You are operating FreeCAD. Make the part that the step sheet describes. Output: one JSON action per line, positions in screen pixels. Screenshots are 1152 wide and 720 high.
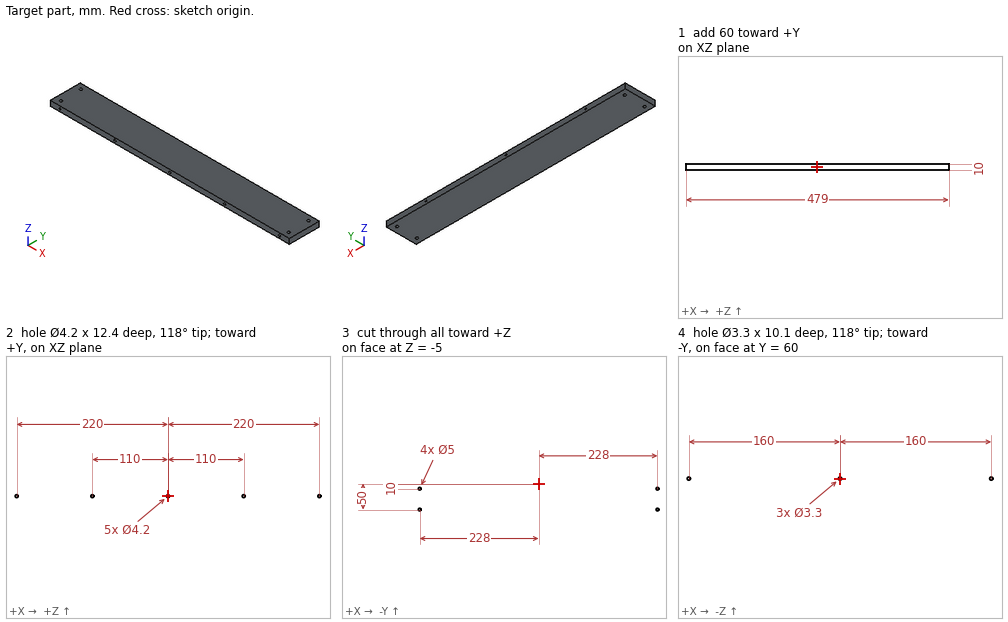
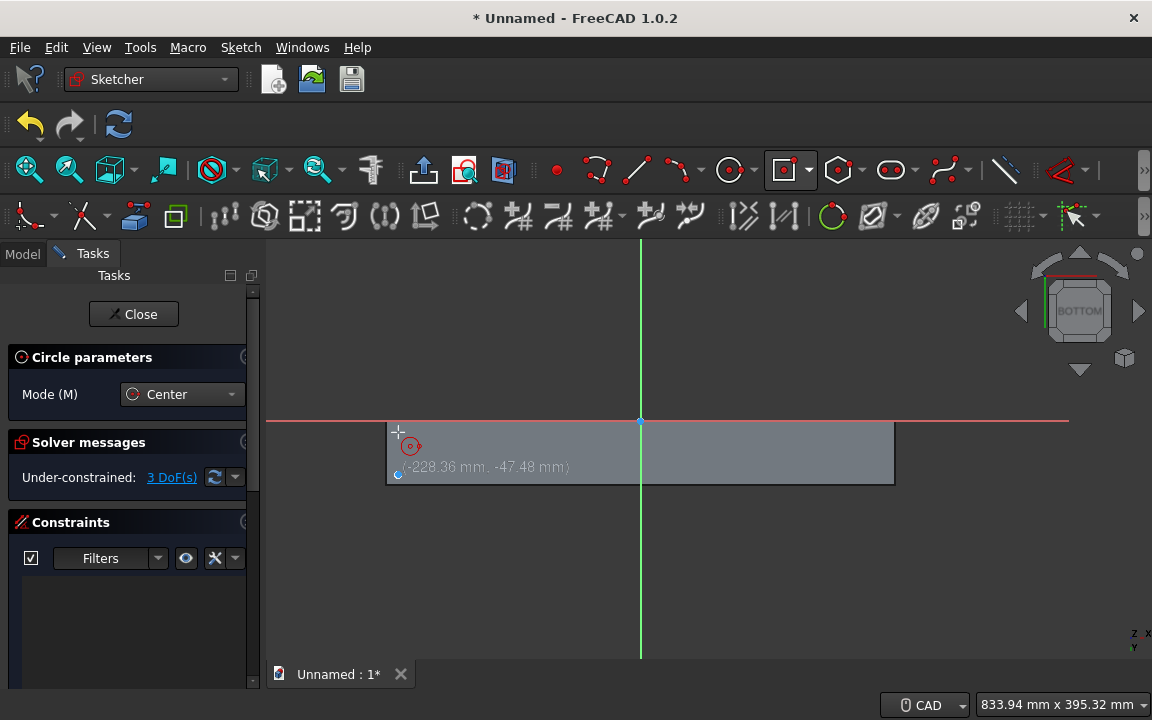
{"action": "scroll", "coordinate": [398, 432], "scroll_direction": "up", "scroll_amount": 3}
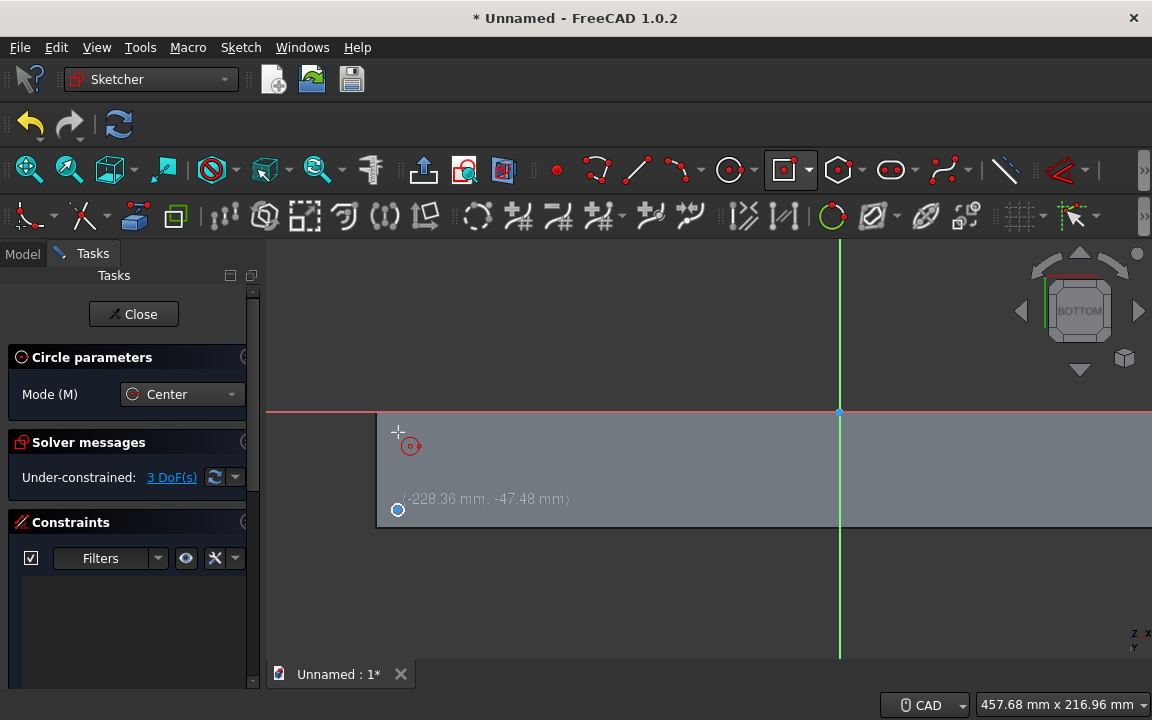
{"action": "left_click", "coordinate": [399, 431]}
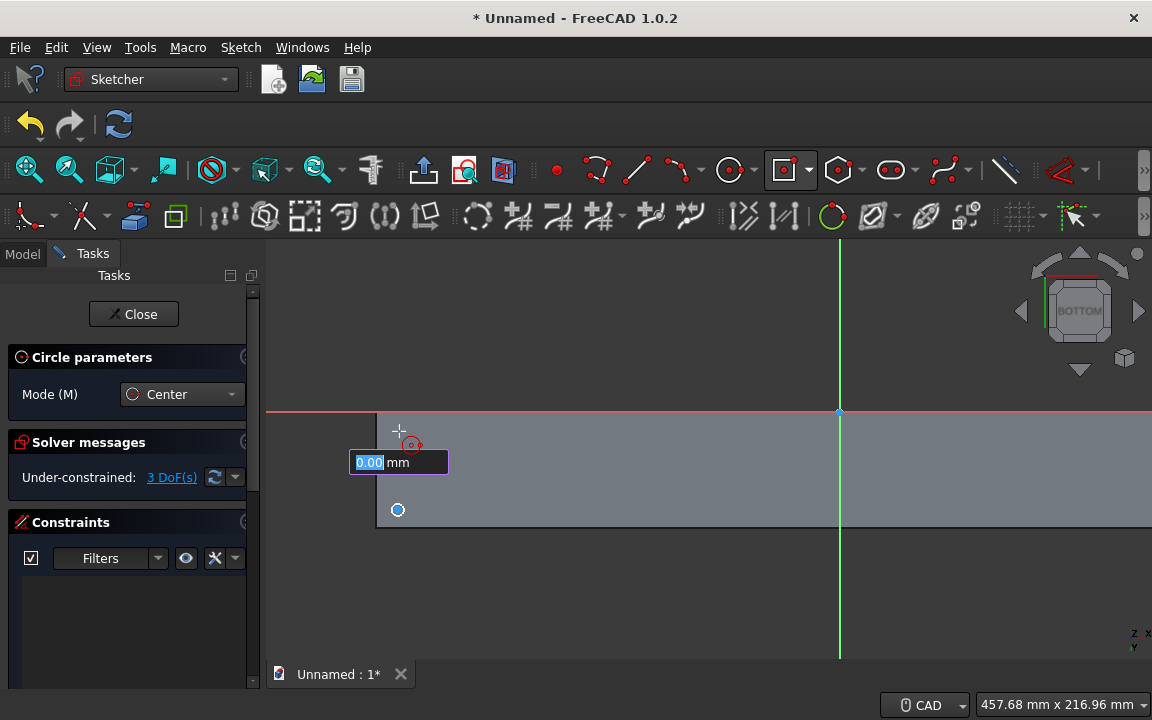
{"action": "scroll", "coordinate": [402, 428], "scroll_direction": "up", "scroll_amount": 6}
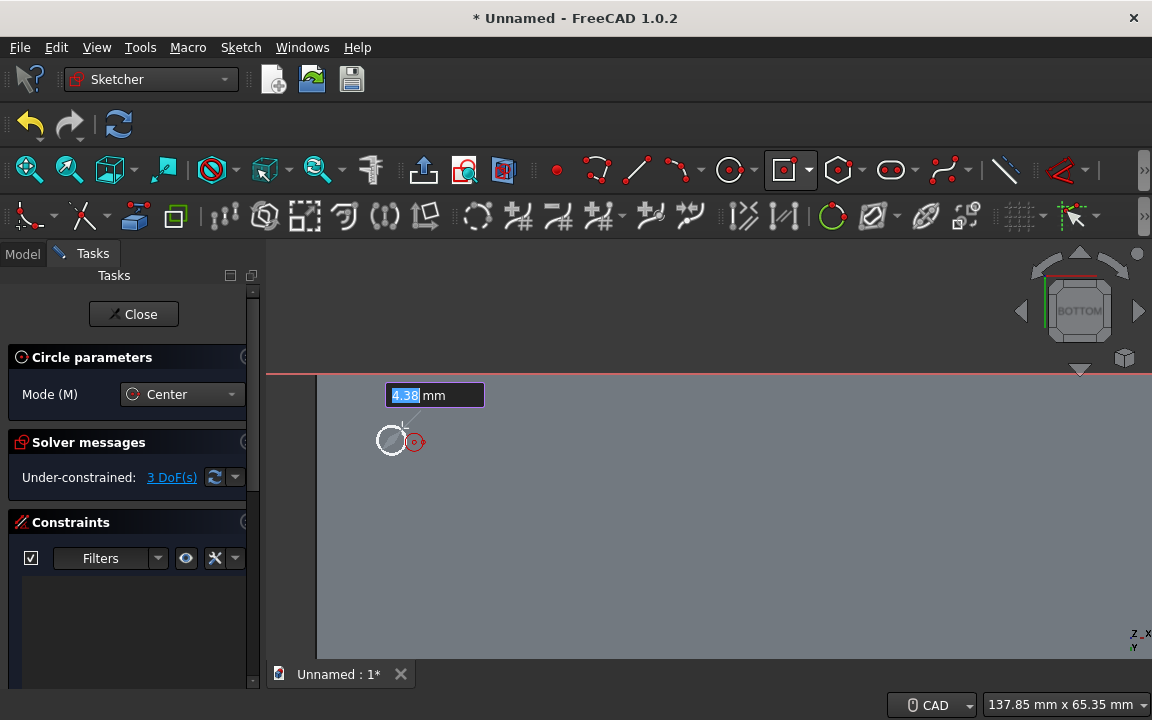
{"action": "left_click", "coordinate": [402, 427]}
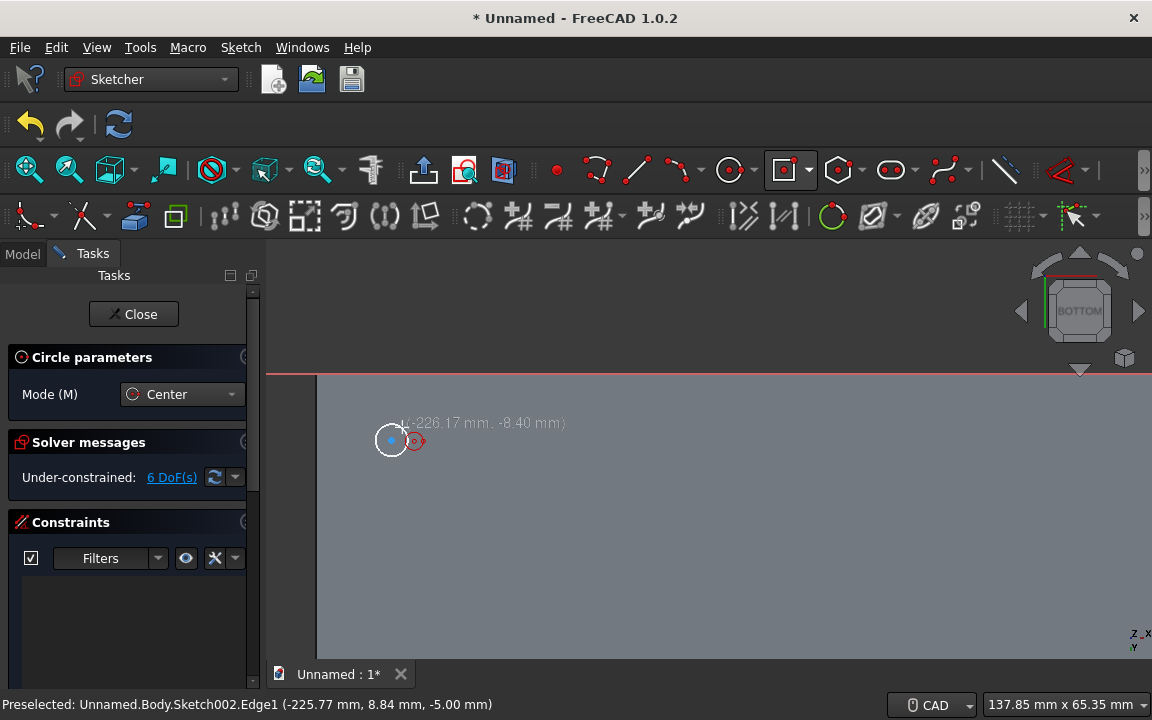
{"action": "scroll", "coordinate": [400, 430], "scroll_direction": "down", "scroll_amount": 9}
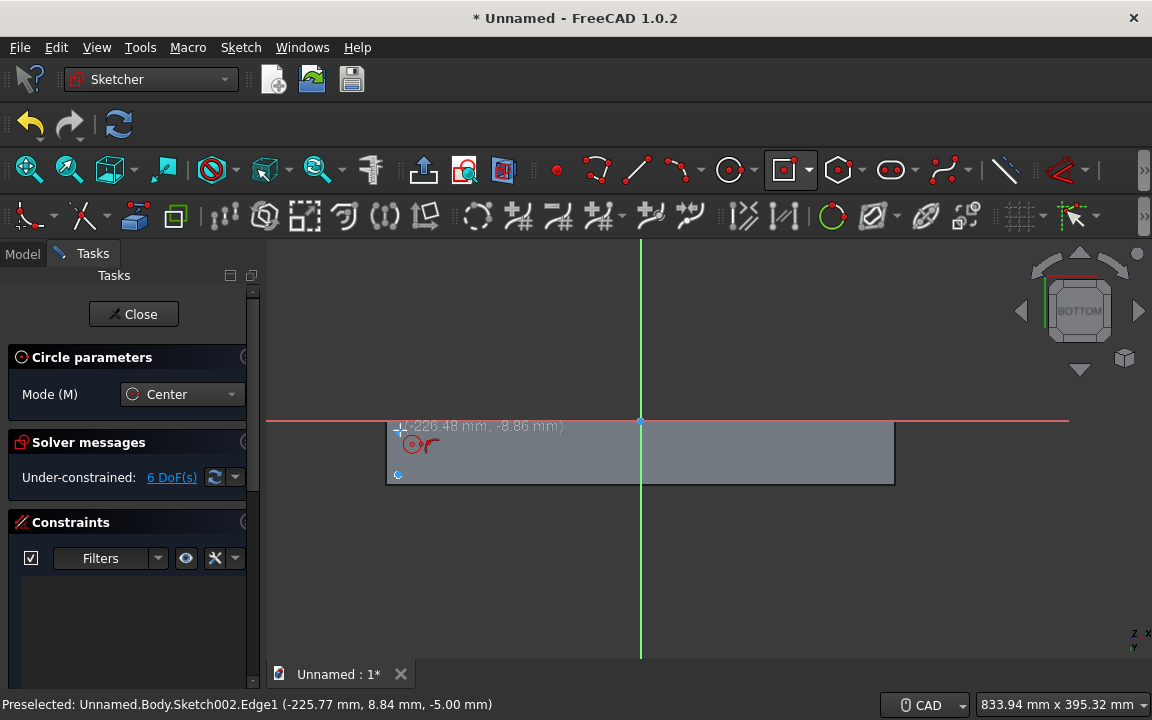
{"action": "scroll", "coordinate": [883, 432], "scroll_direction": "up", "scroll_amount": 11}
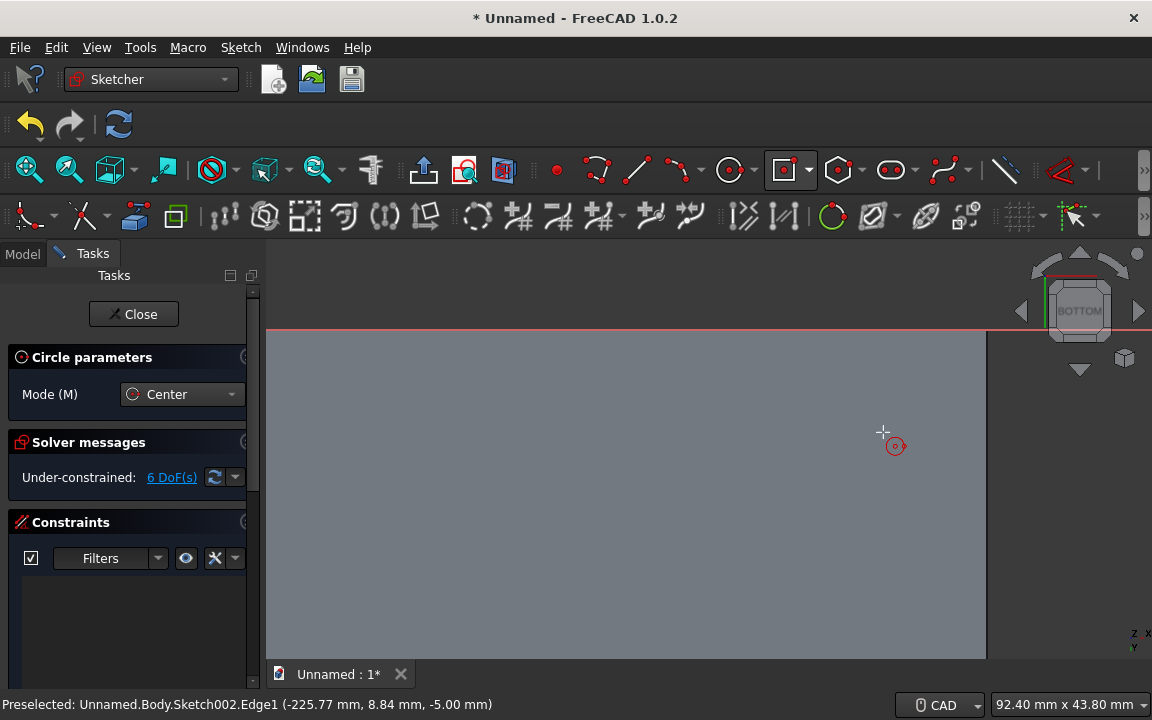
{"action": "scroll", "coordinate": [883, 432], "scroll_direction": "down", "scroll_amount": 11}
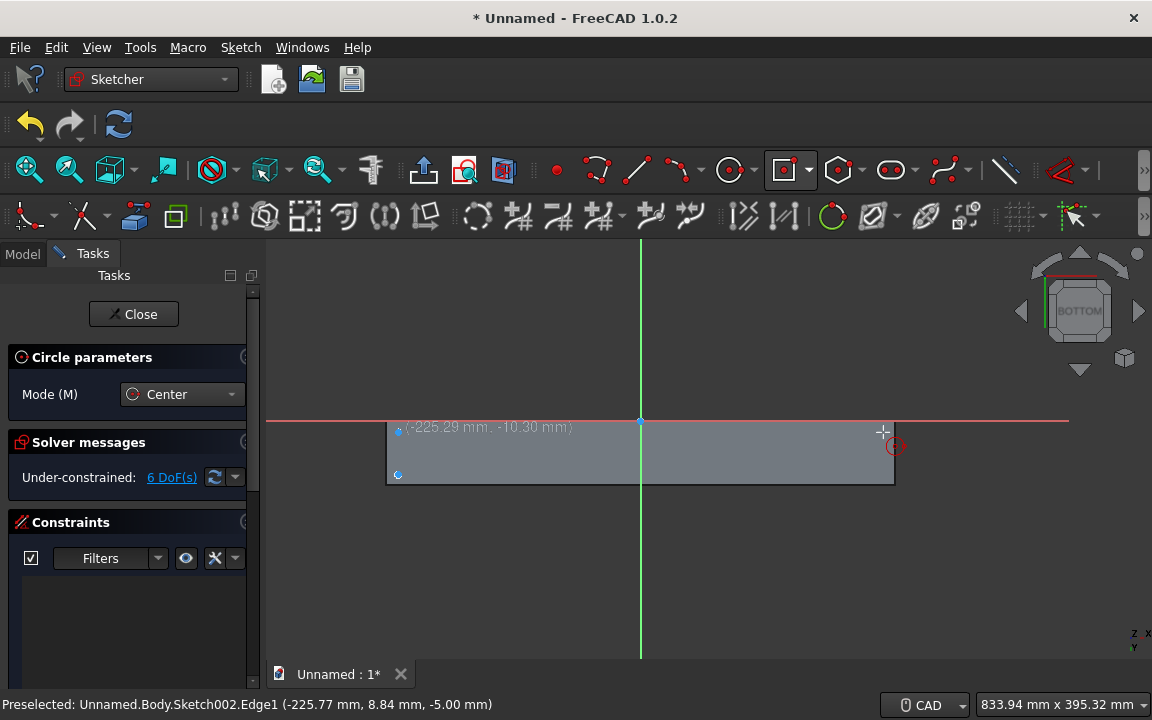
{"action": "scroll", "coordinate": [883, 432], "scroll_direction": "up", "scroll_amount": 3}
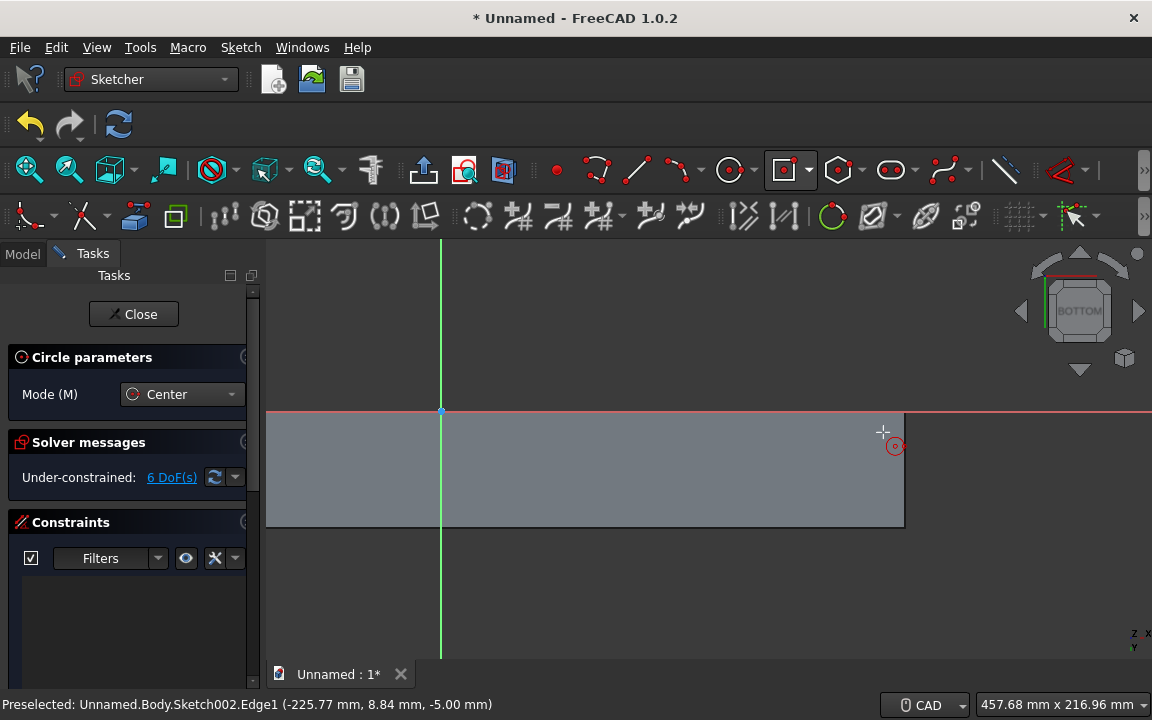
{"action": "left_click", "coordinate": [882, 431]}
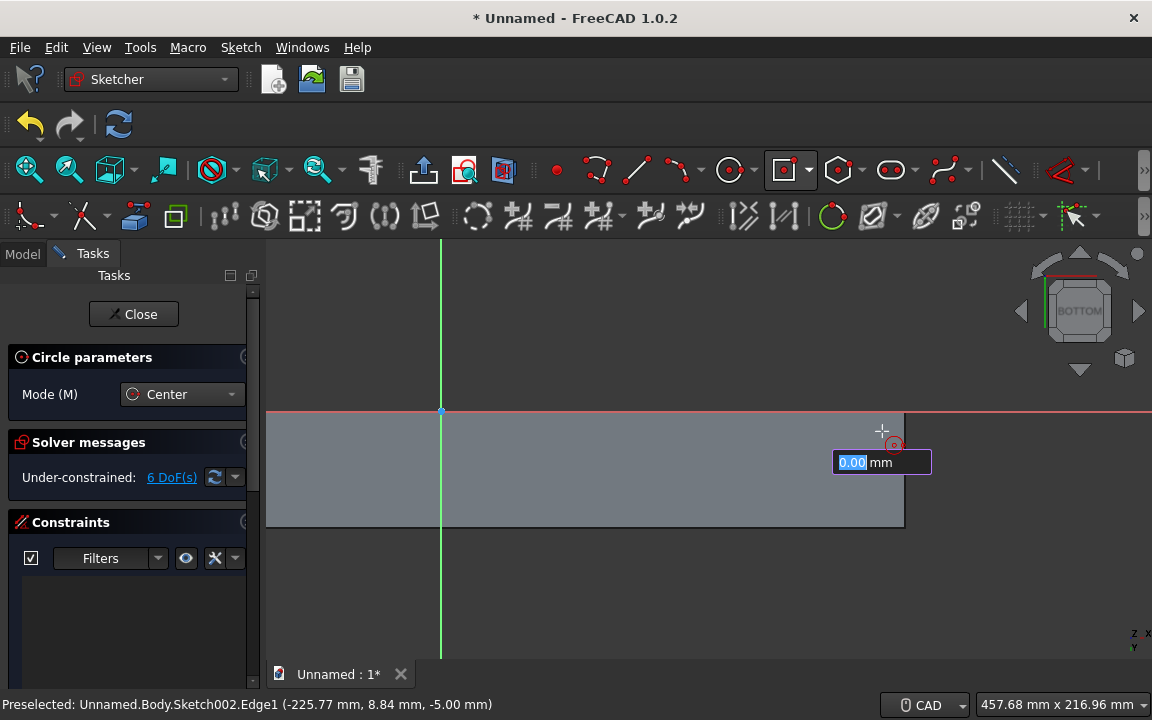
{"action": "scroll", "coordinate": [886, 428], "scroll_direction": "up", "scroll_amount": 6}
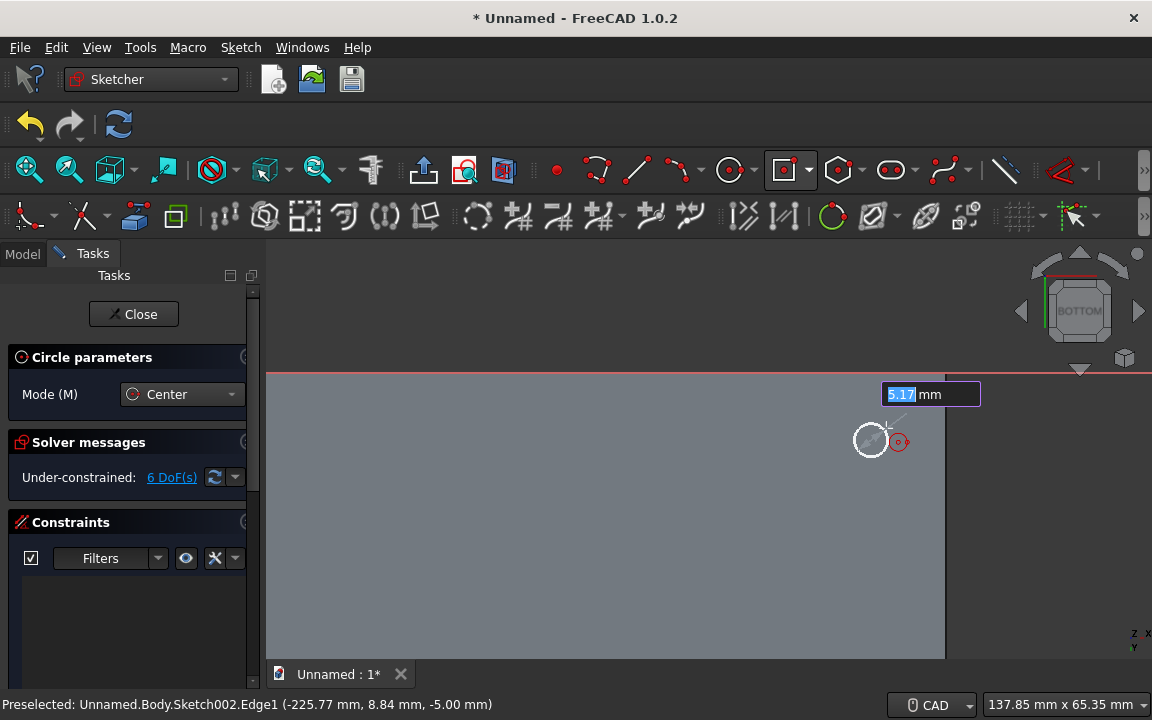
{"action": "left_click", "coordinate": [884, 426]}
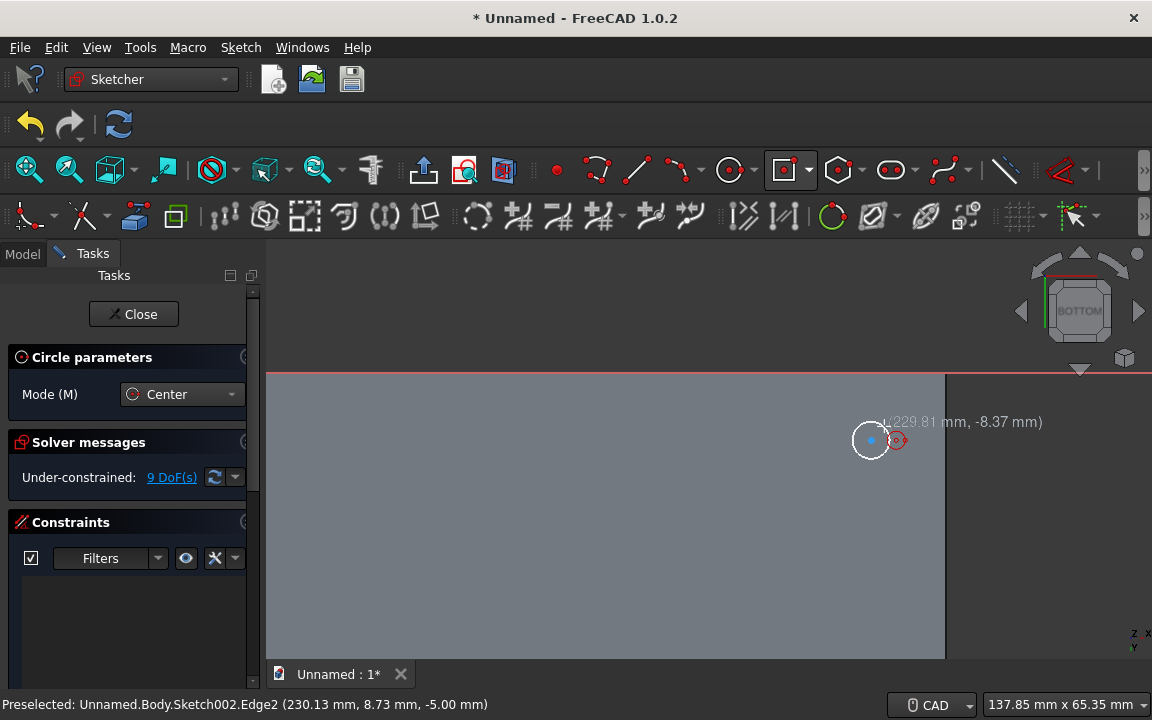
{"action": "scroll", "coordinate": [885, 431], "scroll_direction": "down", "scroll_amount": 9}